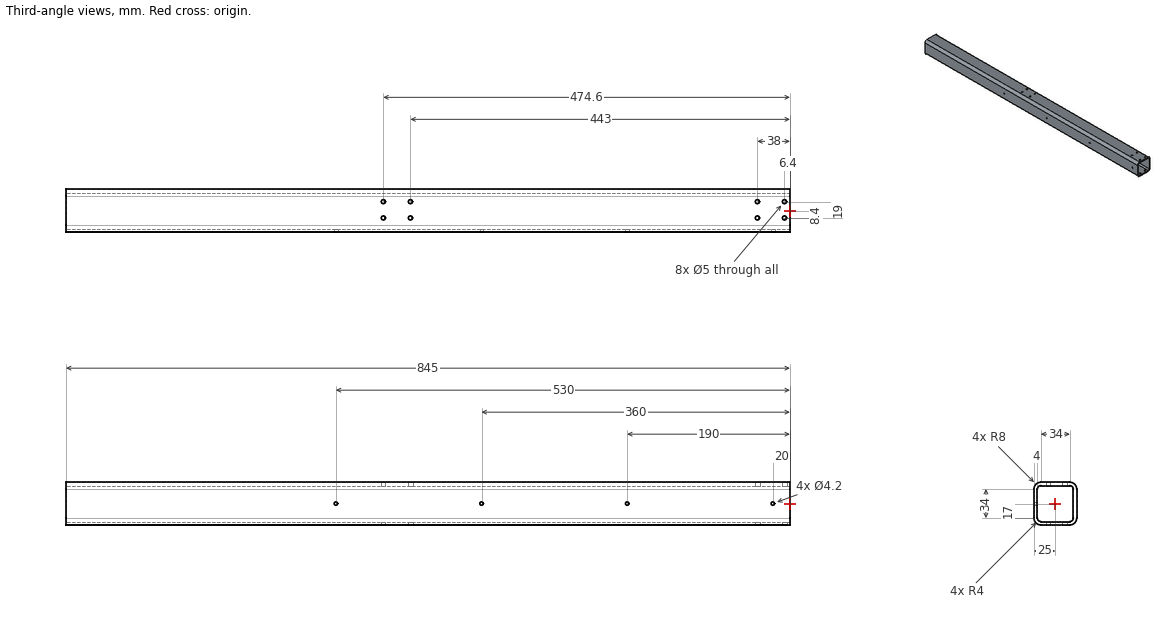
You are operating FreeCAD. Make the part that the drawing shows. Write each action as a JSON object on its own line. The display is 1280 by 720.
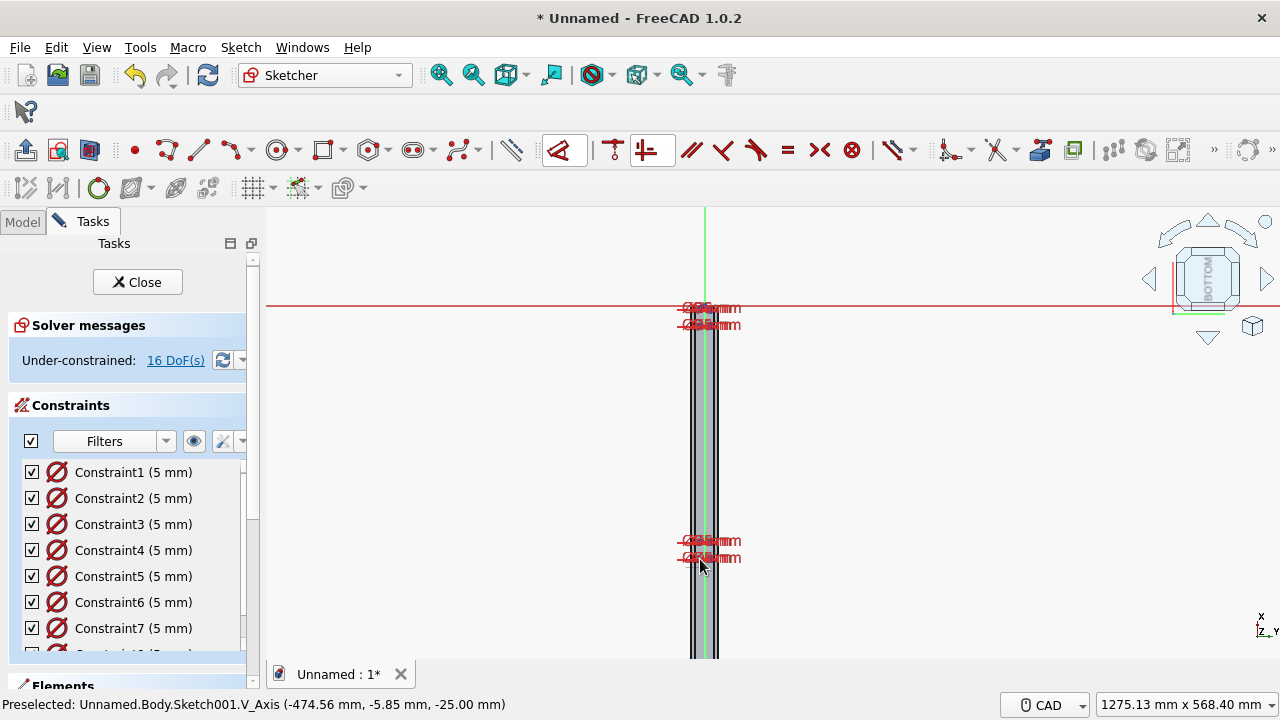
{"action": "scroll", "coordinate": [710, 327], "scroll_direction": "up", "scroll_amount": 4}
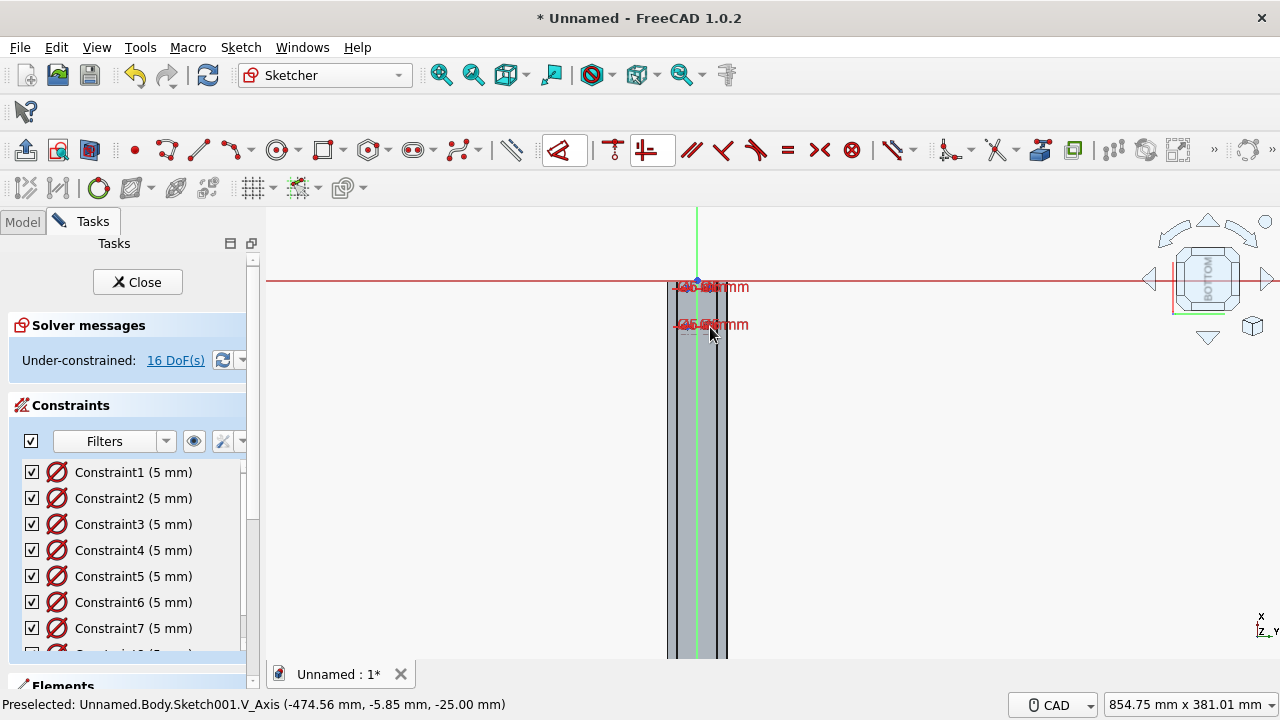
{"action": "left_click", "coordinate": [710, 327]}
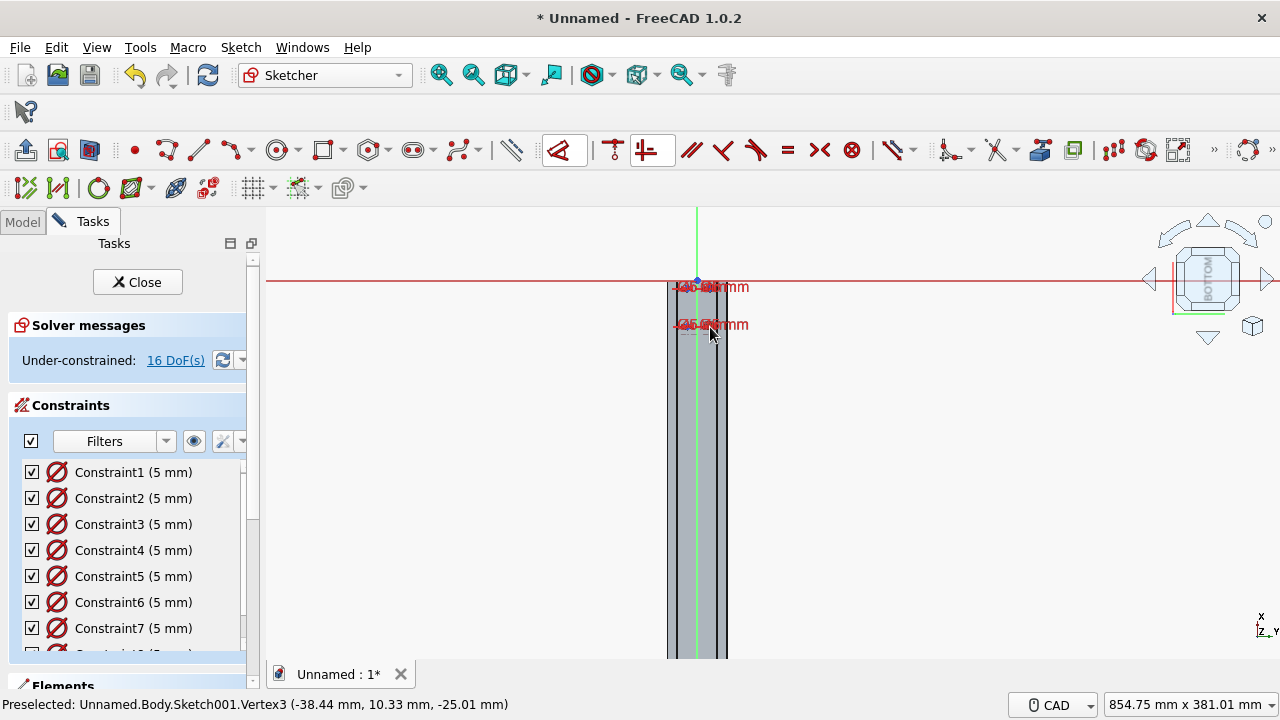
{"action": "left_click", "coordinate": [582, 150]}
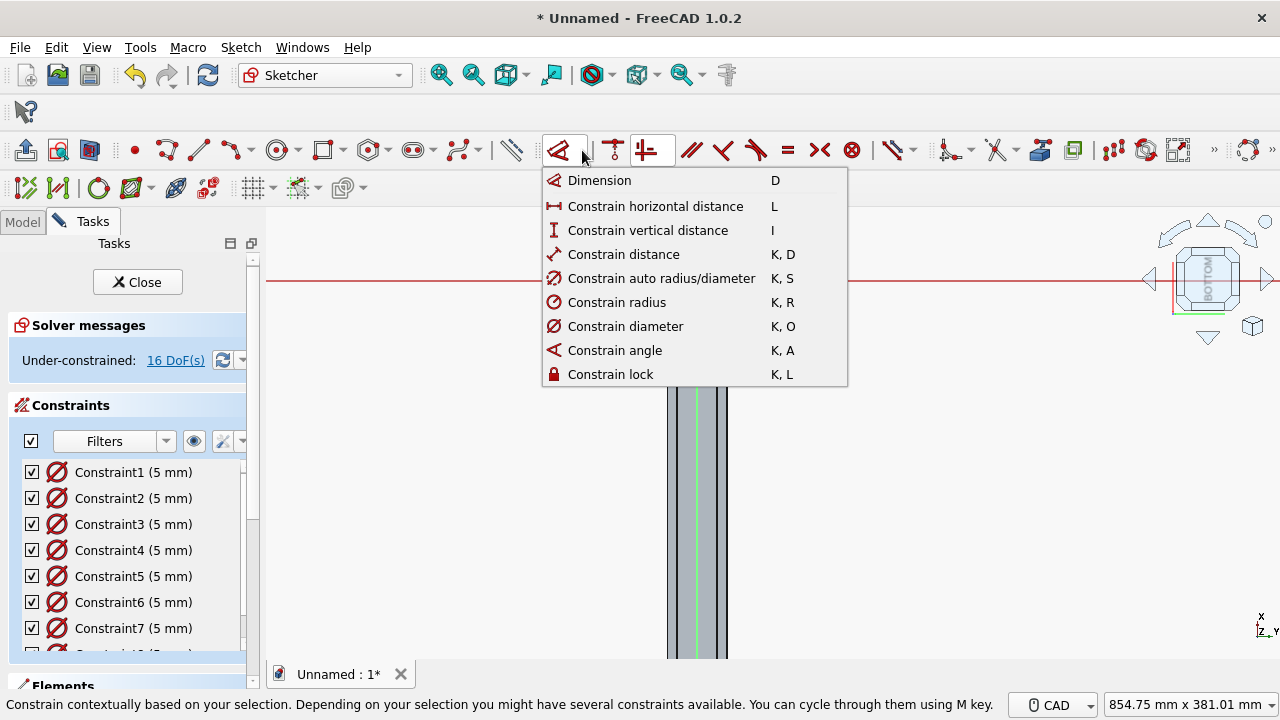
{"action": "left_click", "coordinate": [695, 230]}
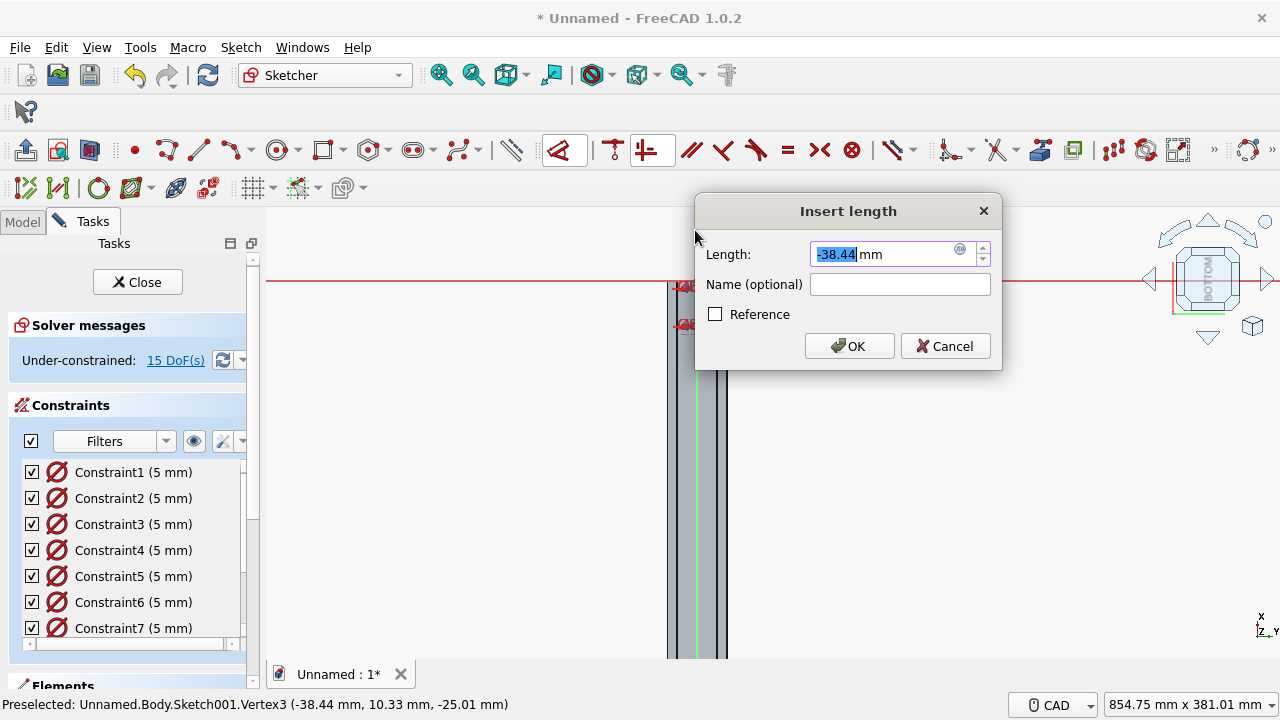
{"action": "type", "text": "-38"}
{"action": "key", "text": "Return"}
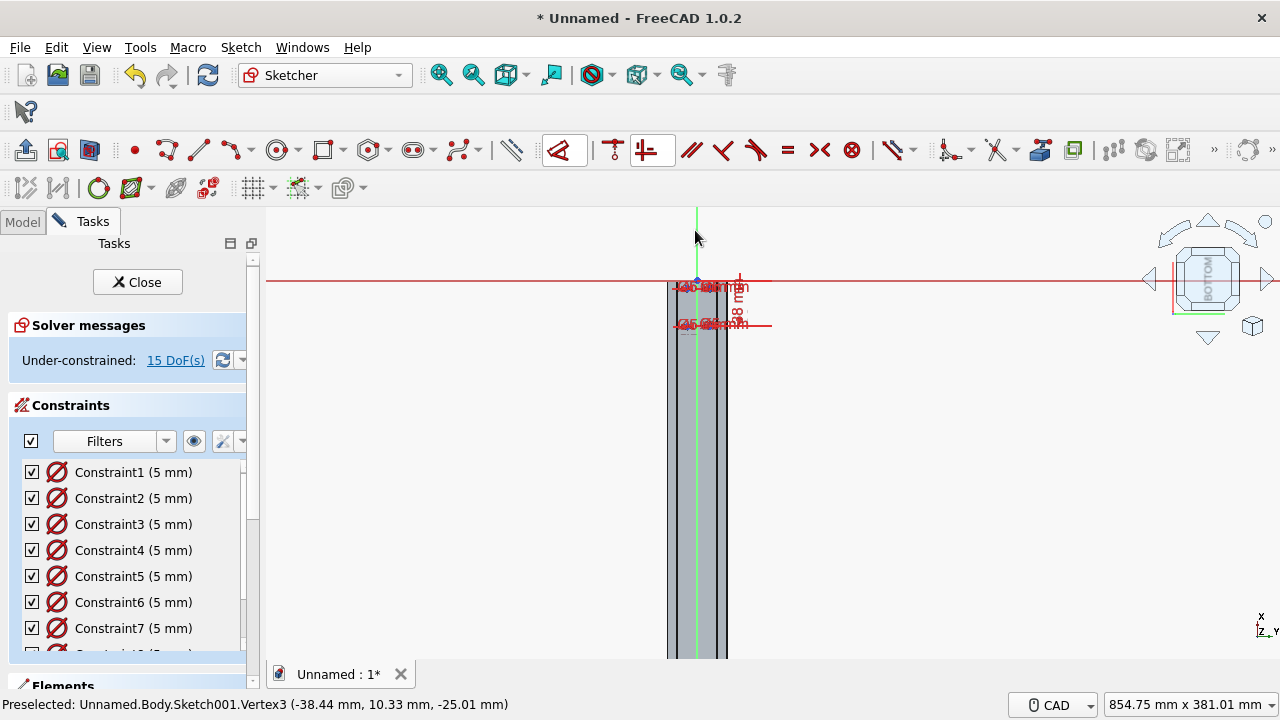
{"action": "left_click", "coordinate": [687, 327]}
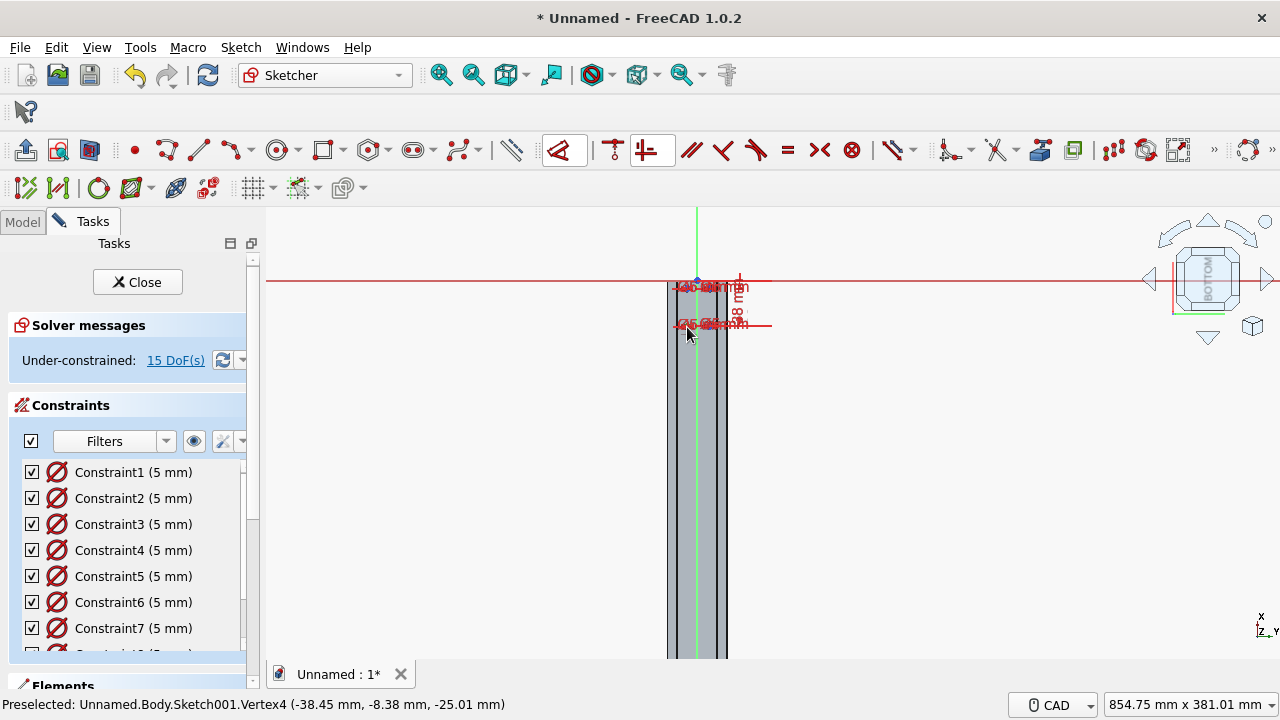
{"action": "left_click", "coordinate": [582, 150]}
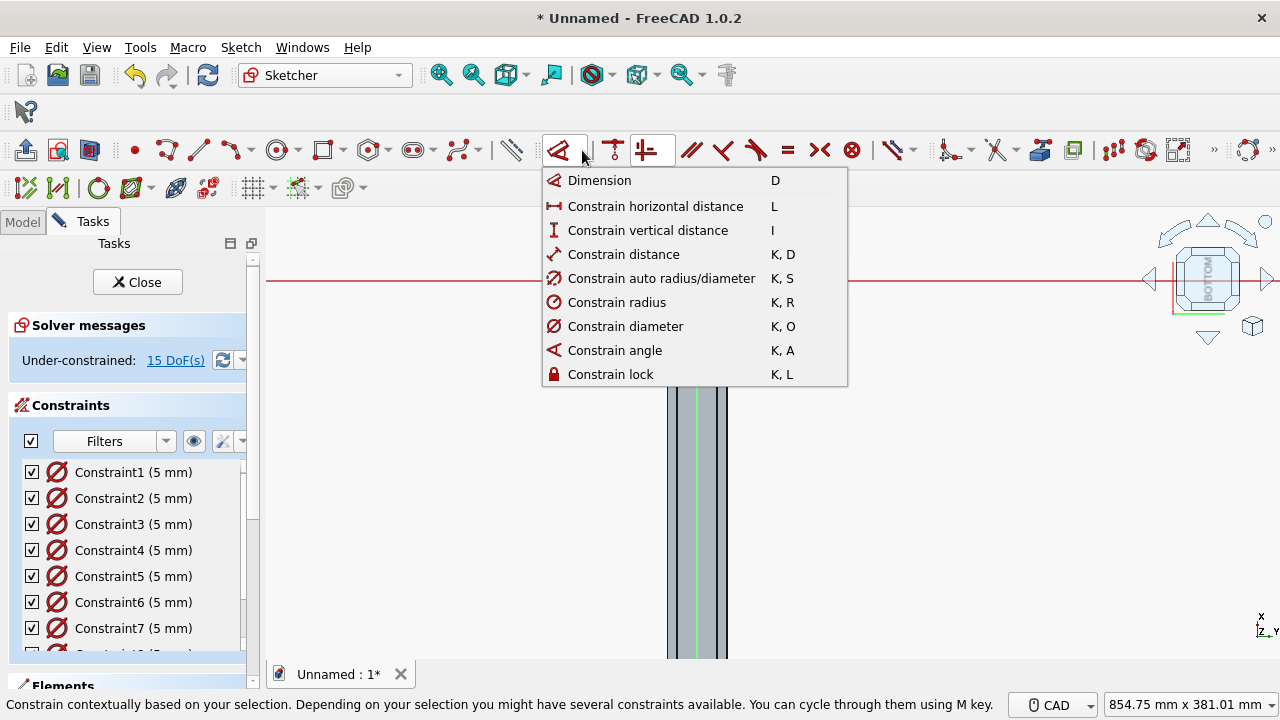
{"action": "left_click", "coordinate": [695, 230]}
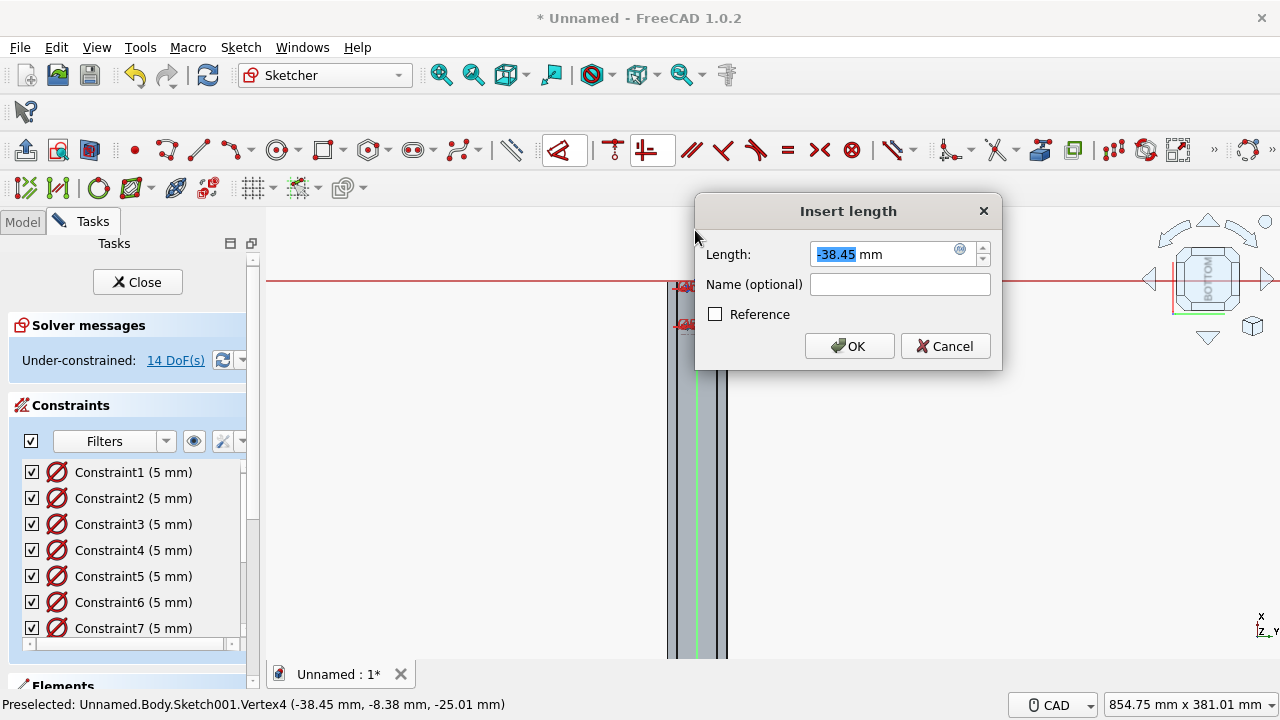
{"action": "type", "text": "-38"}
{"action": "key", "text": "Return"}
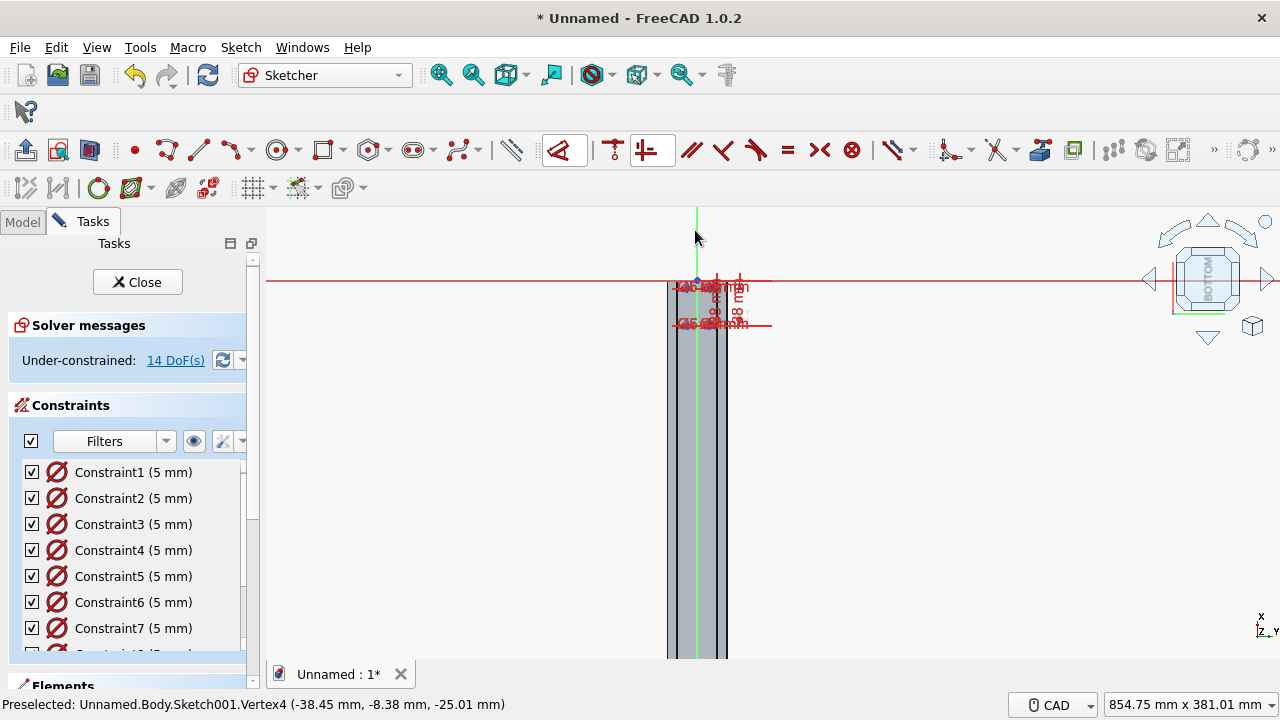
{"action": "scroll", "coordinate": [710, 289], "scroll_direction": "up", "scroll_amount": 9}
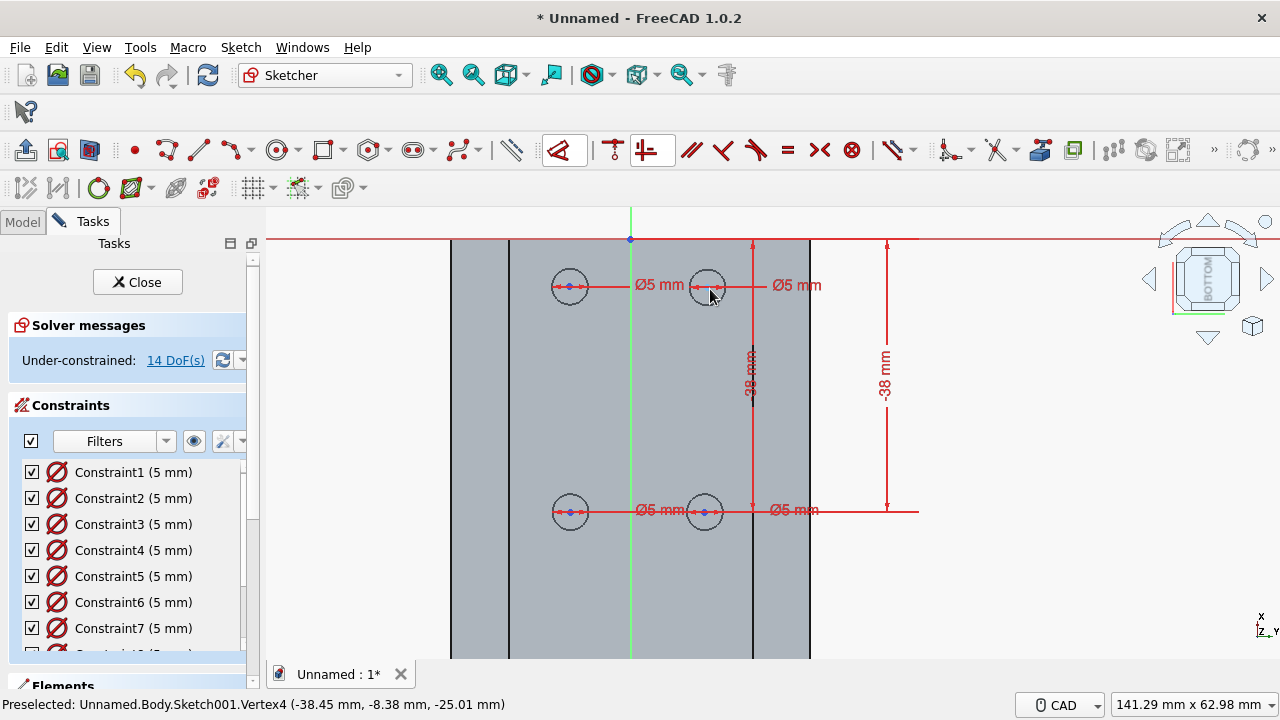
{"action": "left_click", "coordinate": [707, 287]}